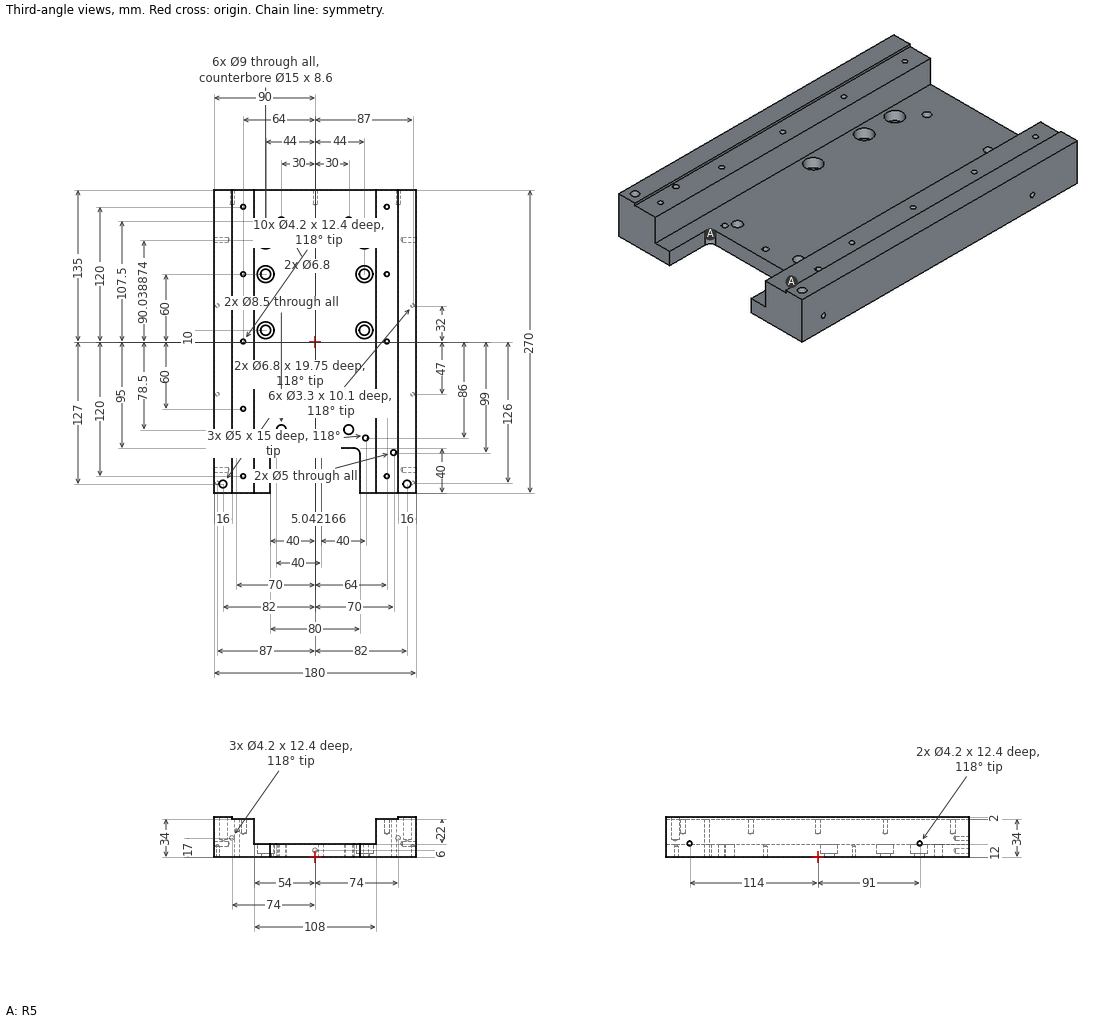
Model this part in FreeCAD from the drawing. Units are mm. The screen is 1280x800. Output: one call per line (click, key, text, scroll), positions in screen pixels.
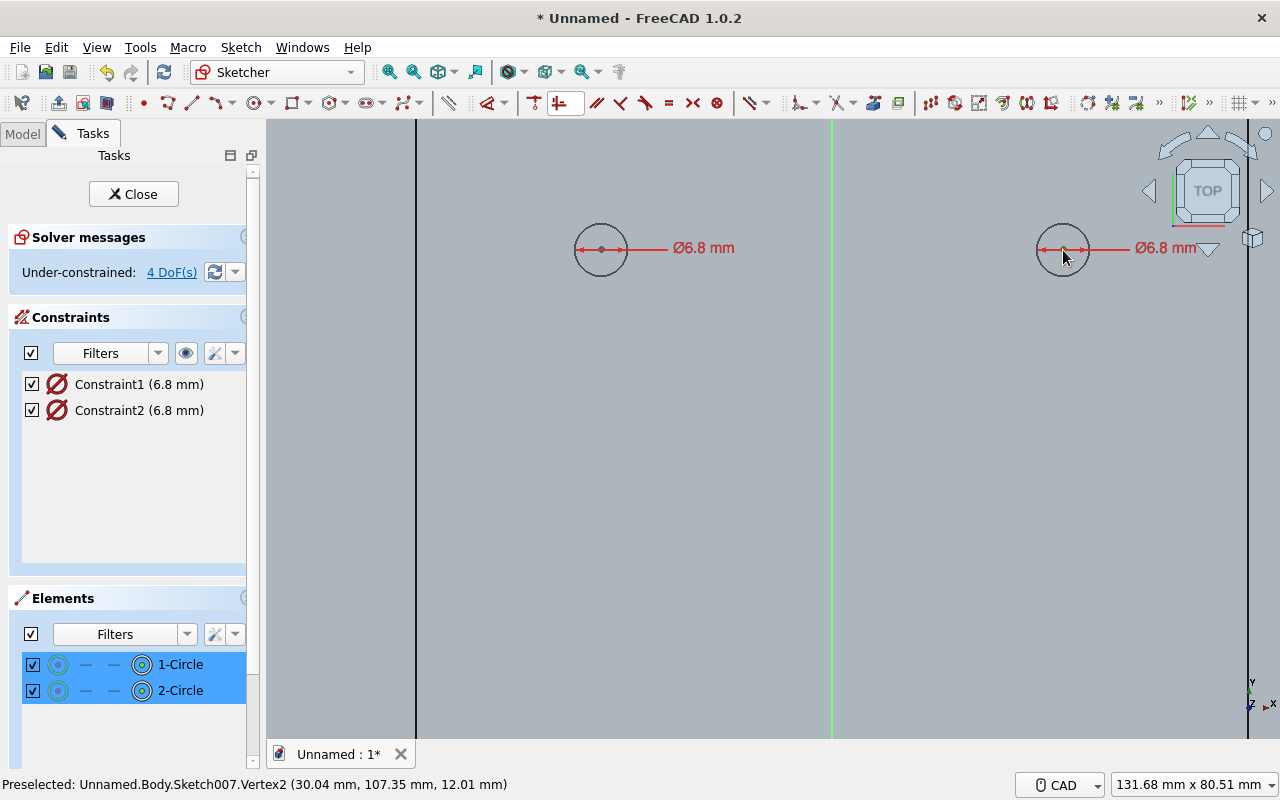
key(h)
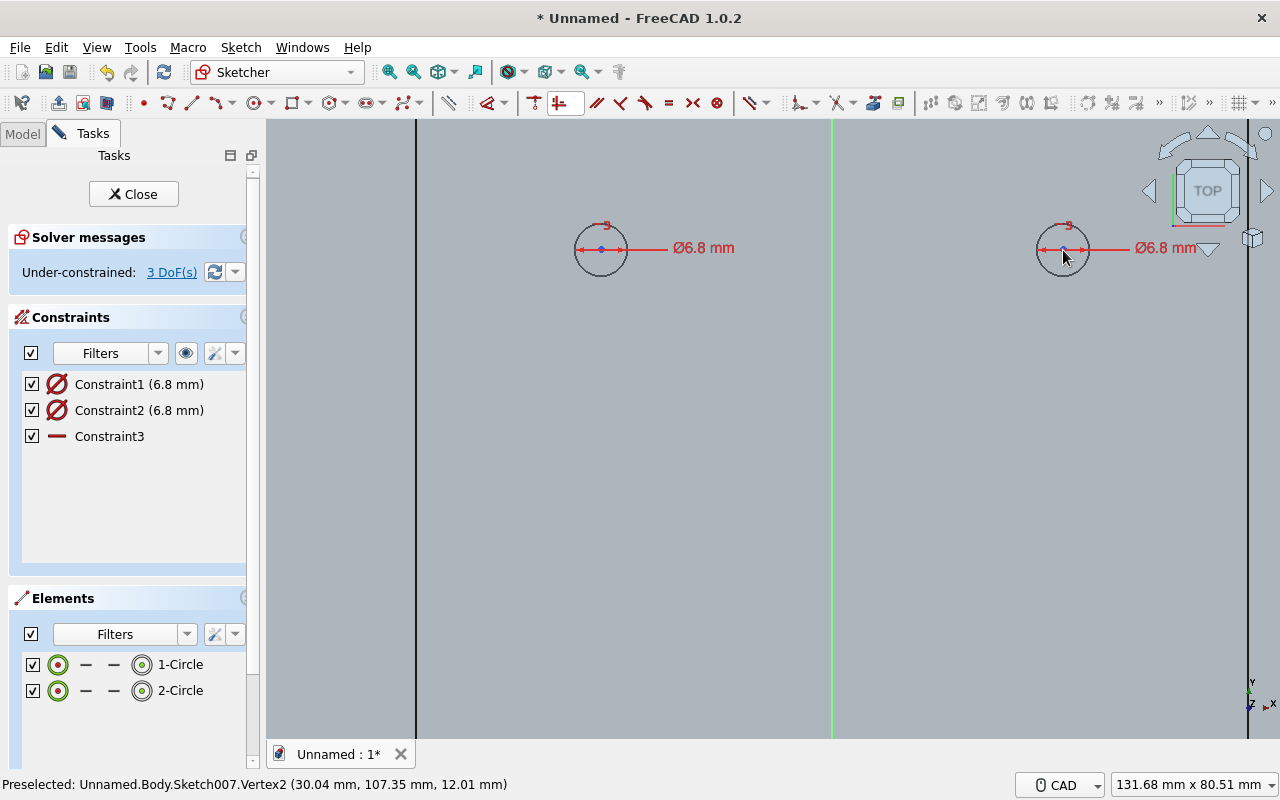
click(488, 104)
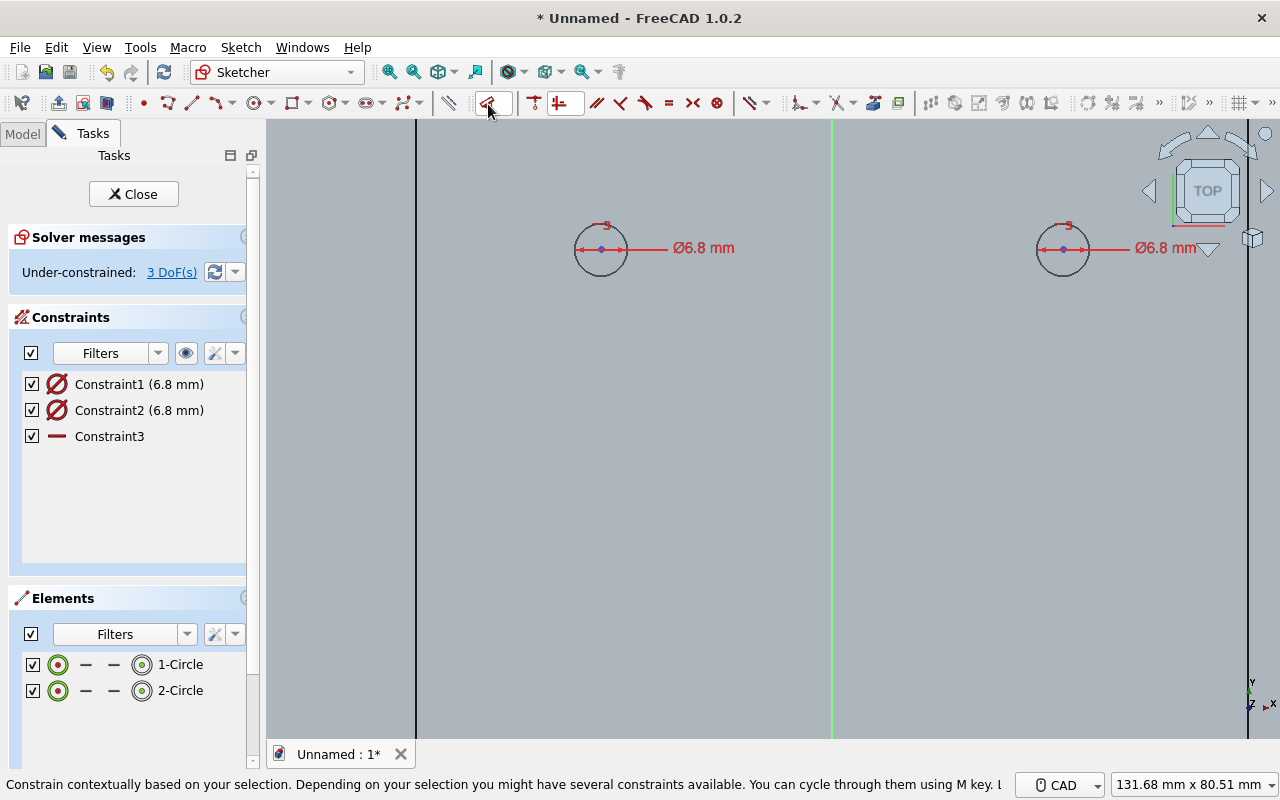
click(601, 250)
click(716, 216)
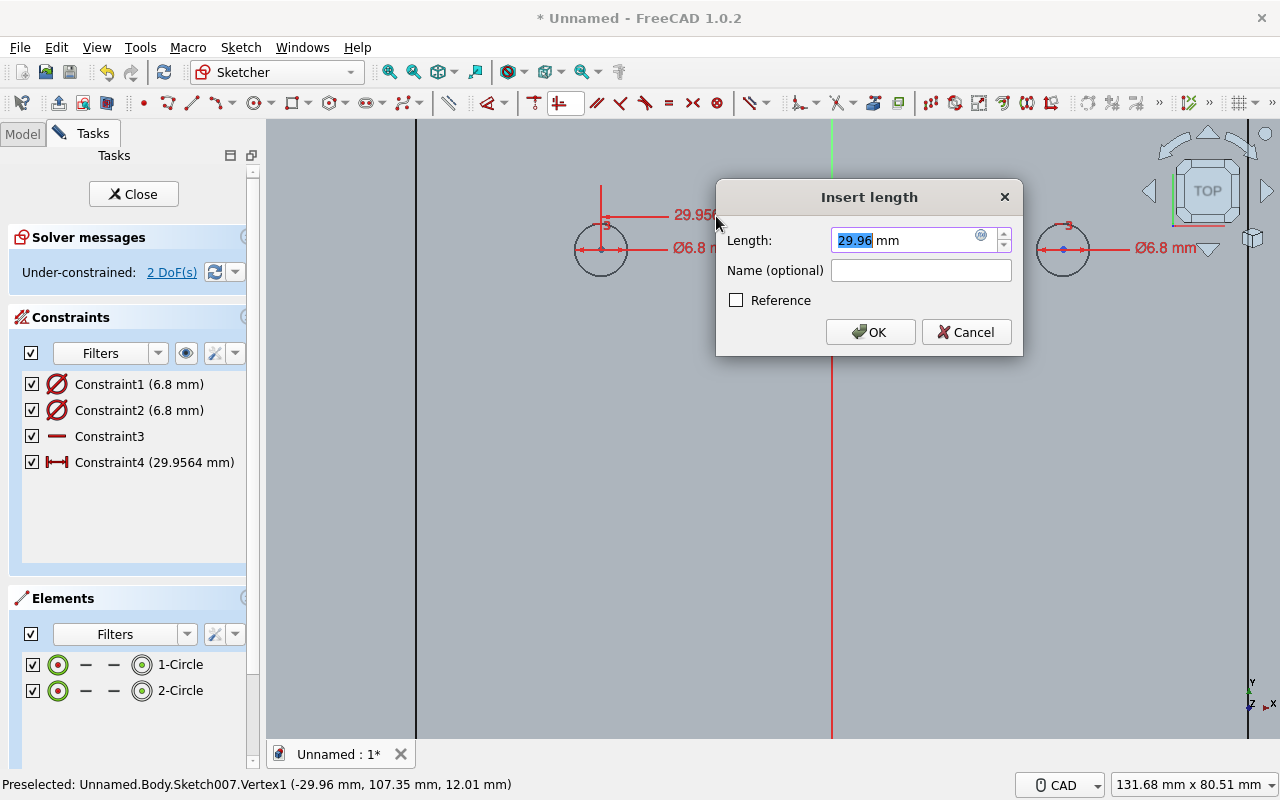
text(30)
key(Return)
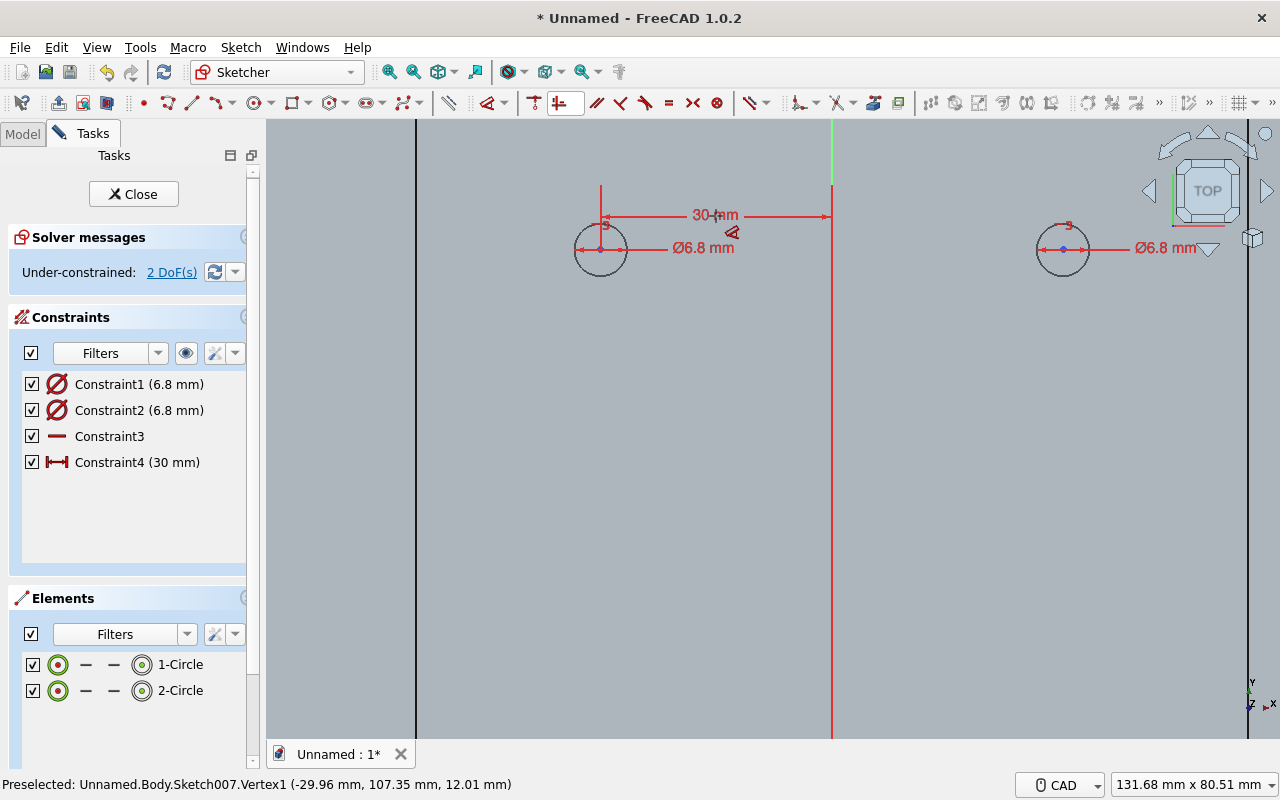
click(1063, 250)
click(947, 216)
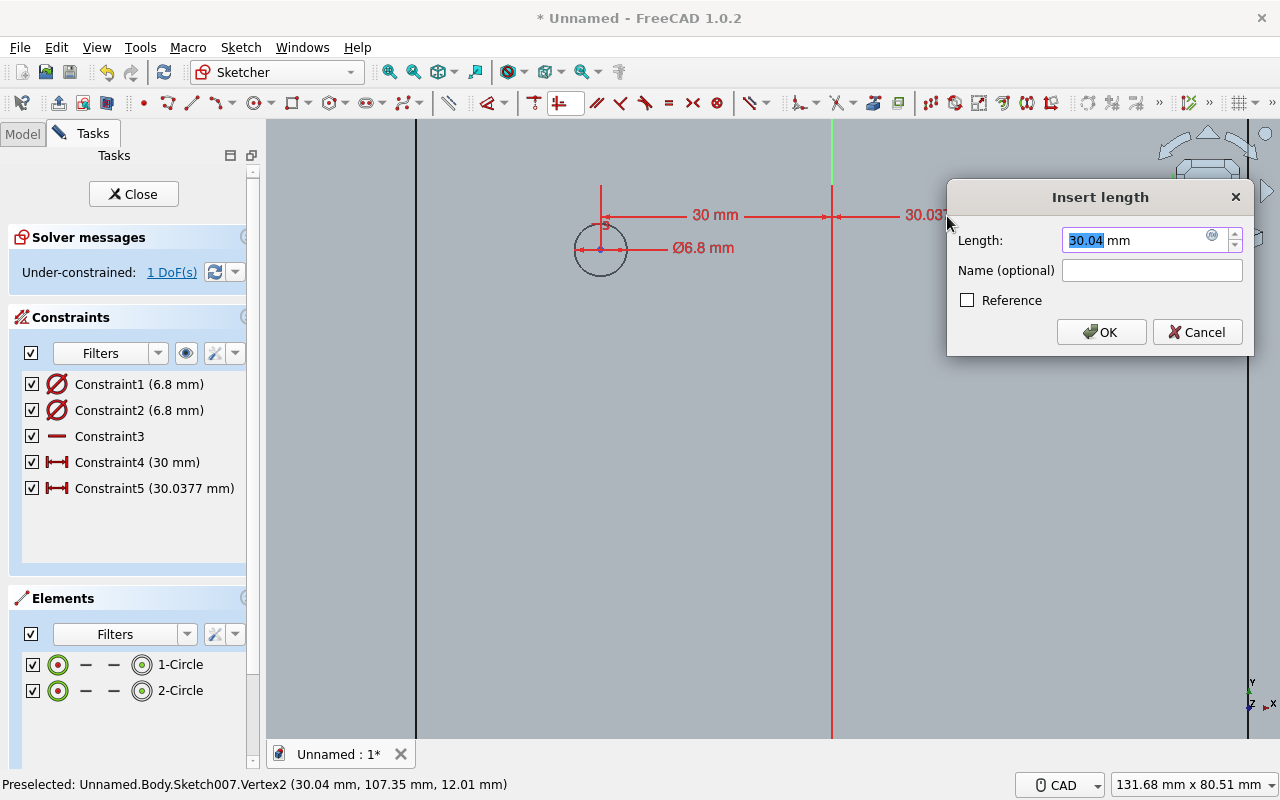
text(30)
key(Return)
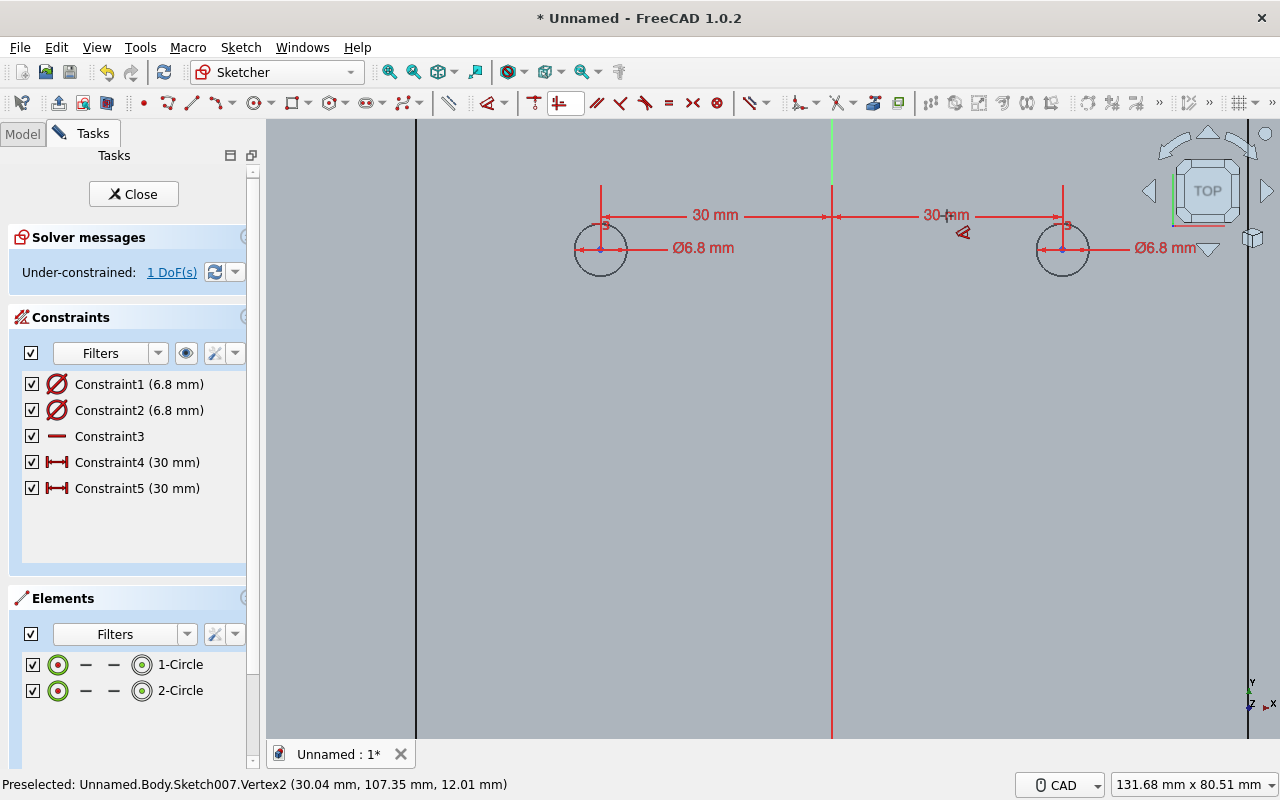
click(601, 250)
click(567, 480)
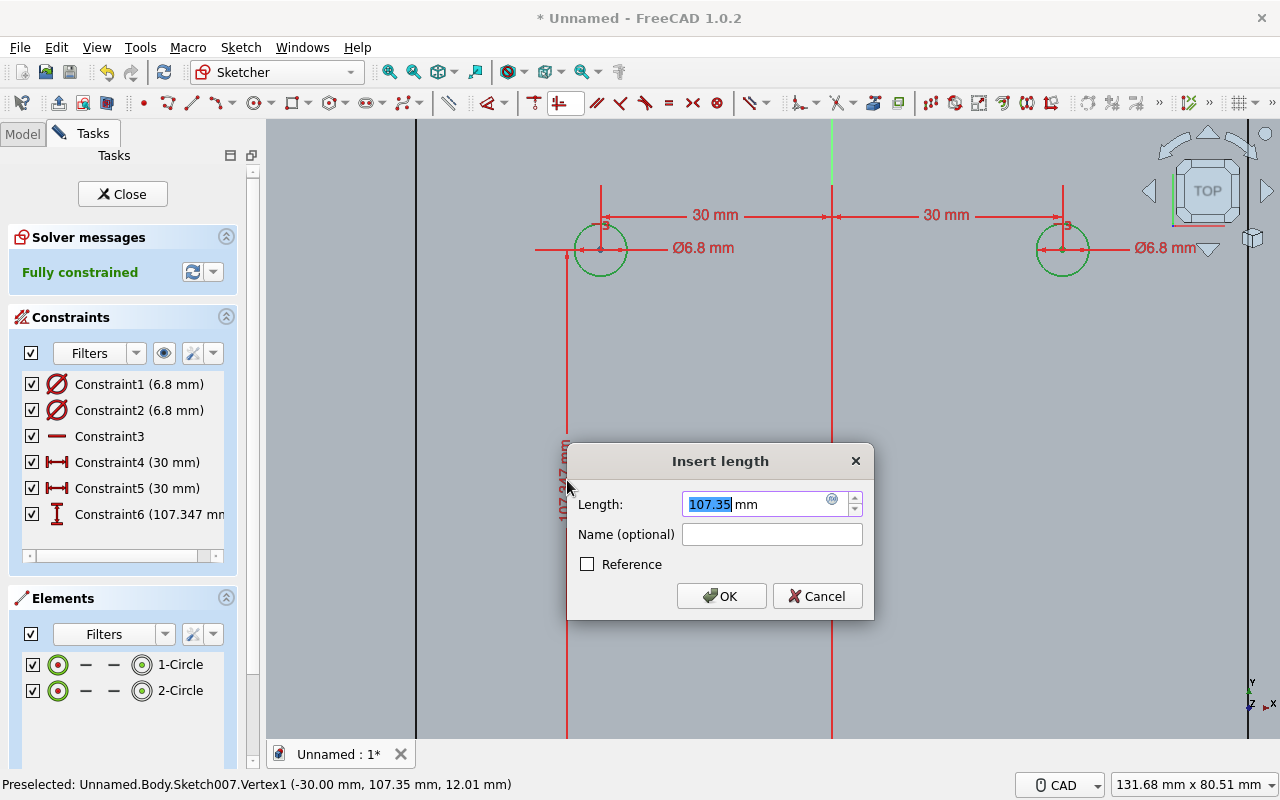
text(107.5)
key(Return)
key(Escape)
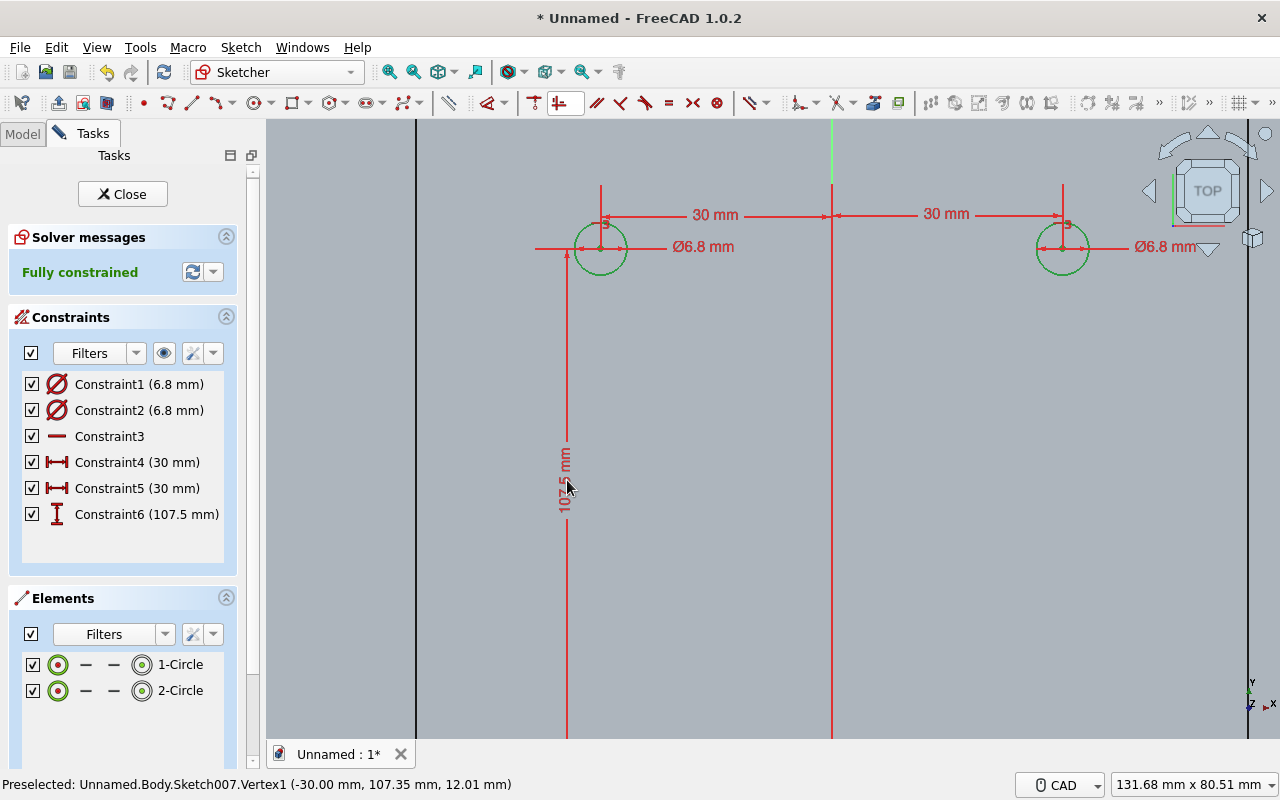
click(123, 194)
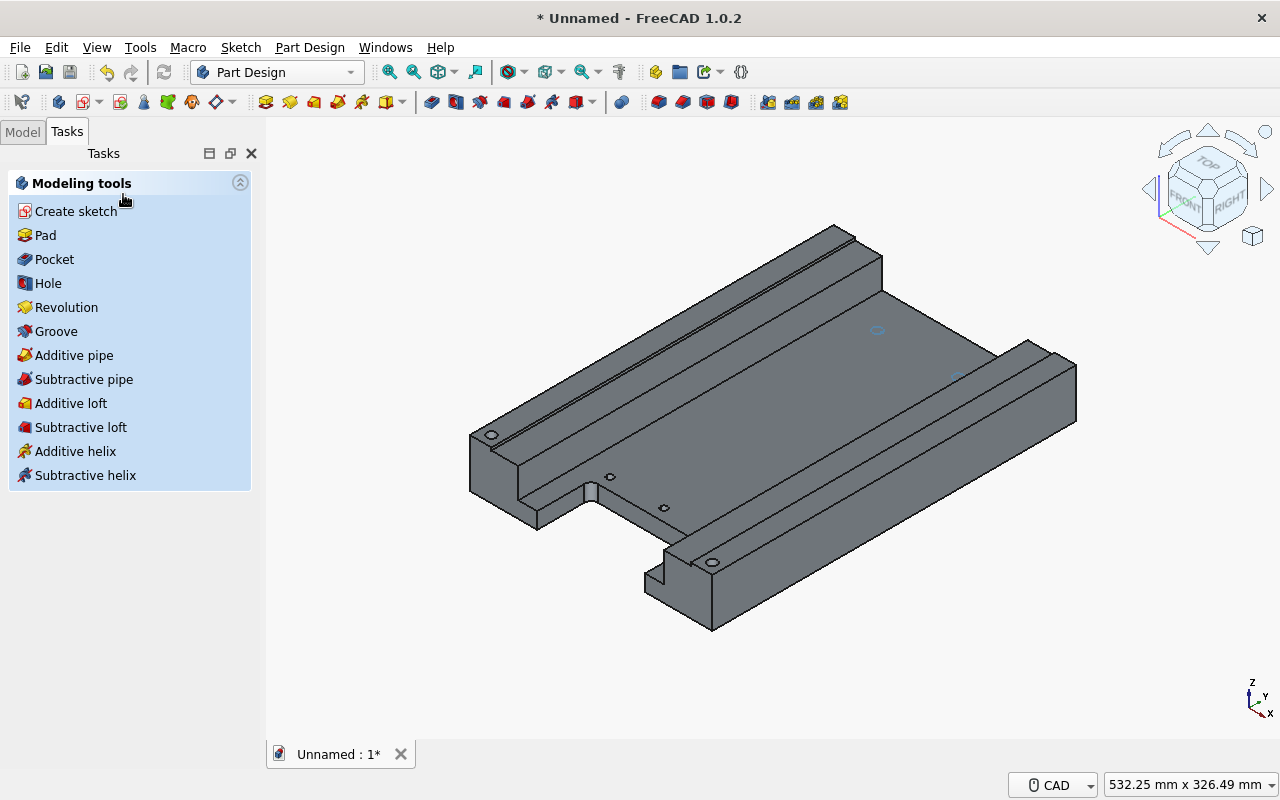
click(432, 102)